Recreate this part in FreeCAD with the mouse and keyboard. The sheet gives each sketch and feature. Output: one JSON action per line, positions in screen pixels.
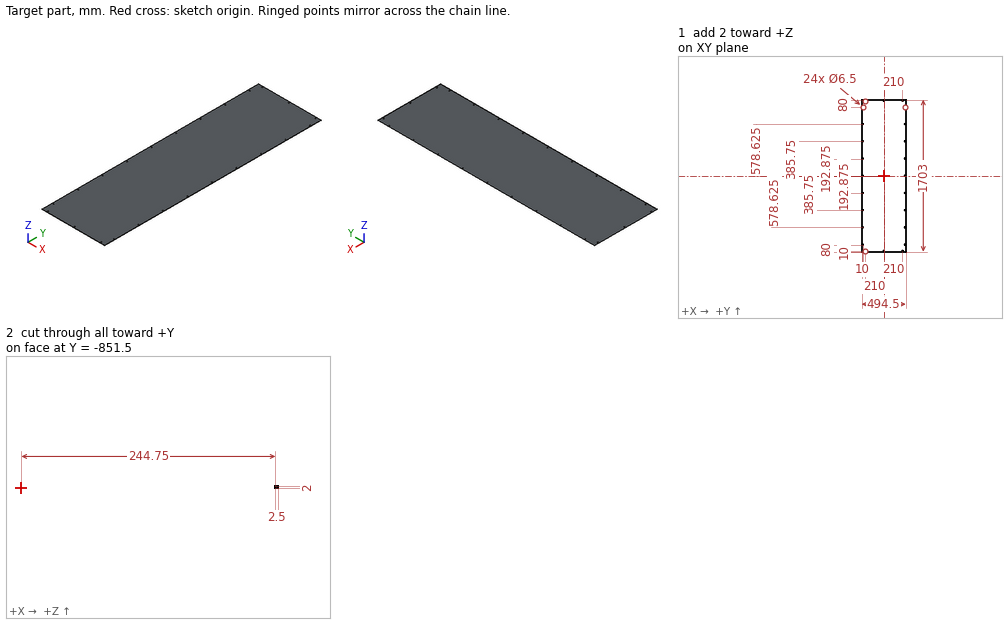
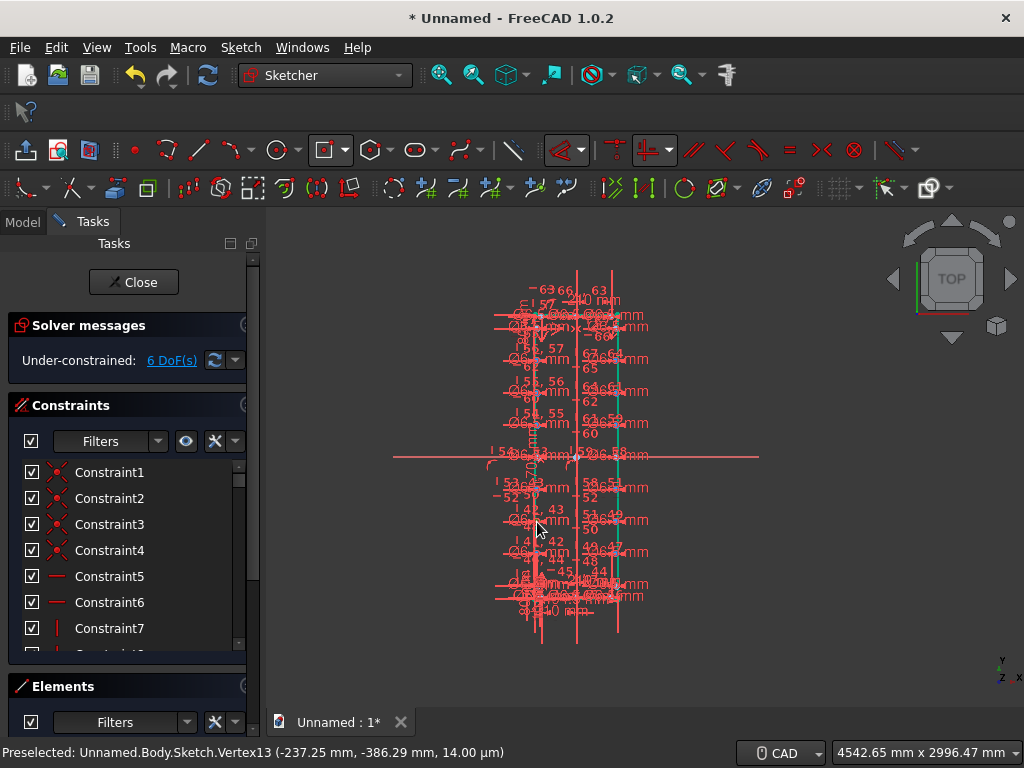
{"action": "left_click", "coordinate": [584, 150]}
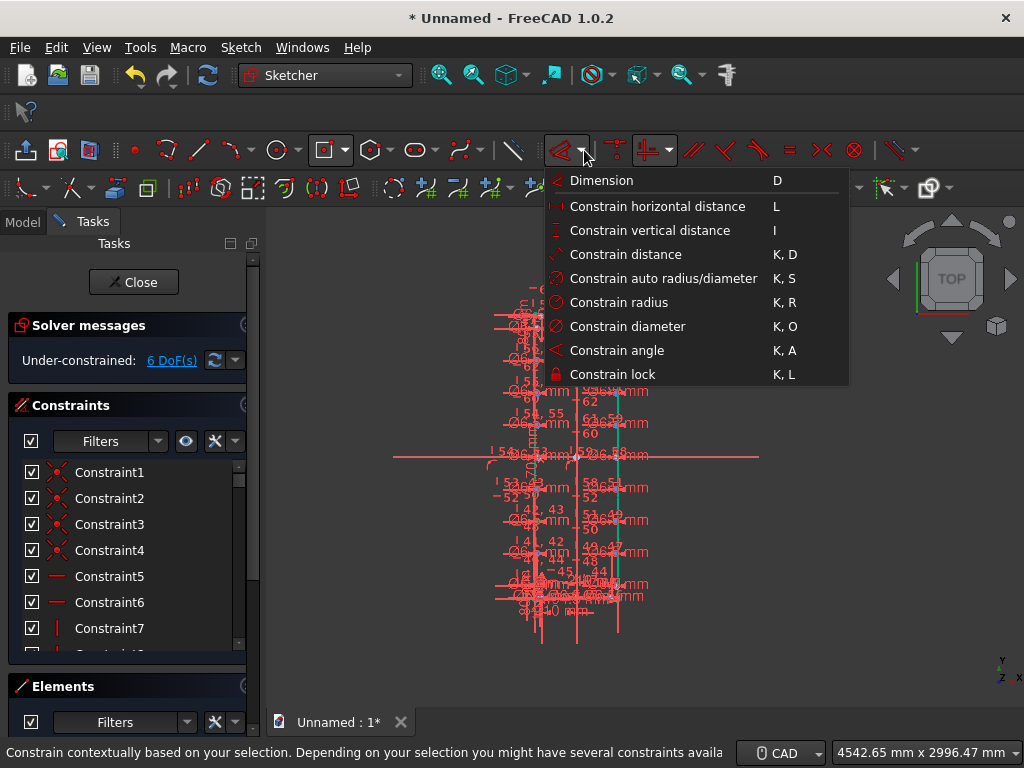
{"action": "left_click", "coordinate": [697, 230]}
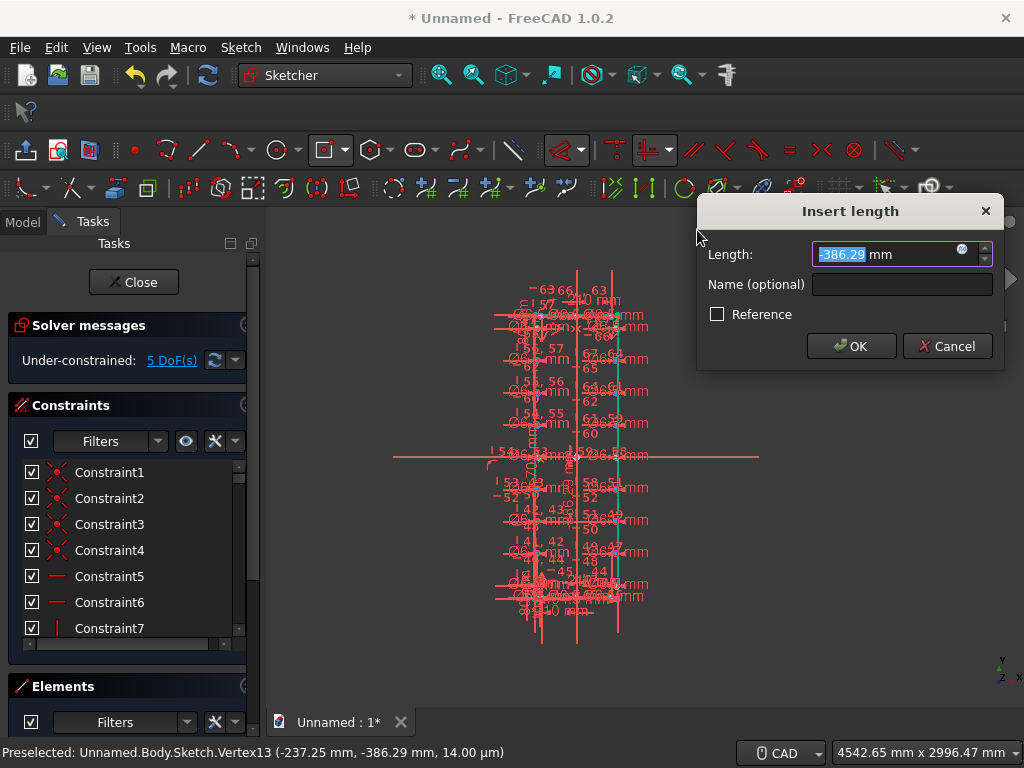
{"action": "type", "text": "-385.75"}
{"action": "key", "text": "Return"}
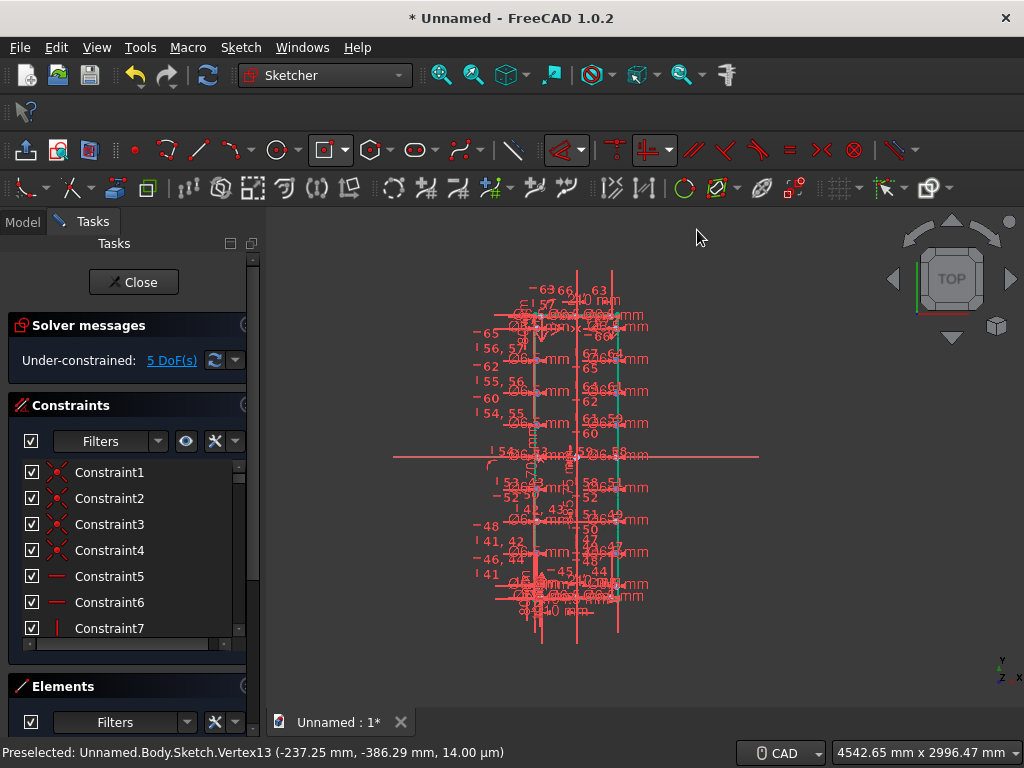
{"action": "left_click", "coordinate": [537, 393]}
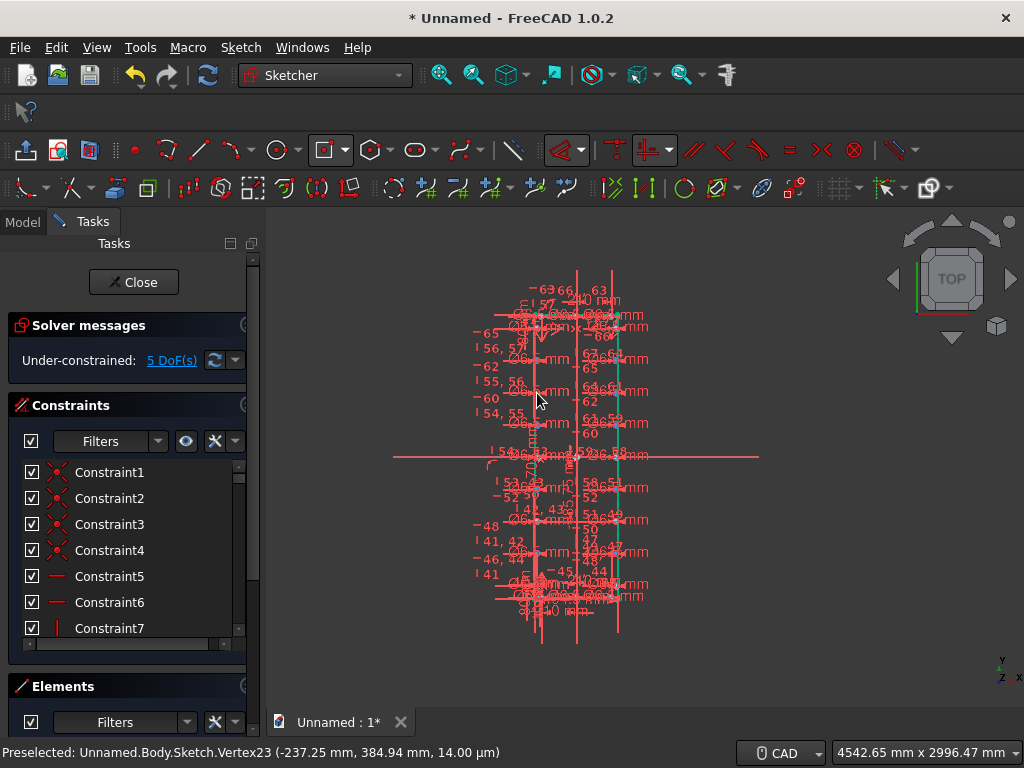
{"action": "key", "text": "i"}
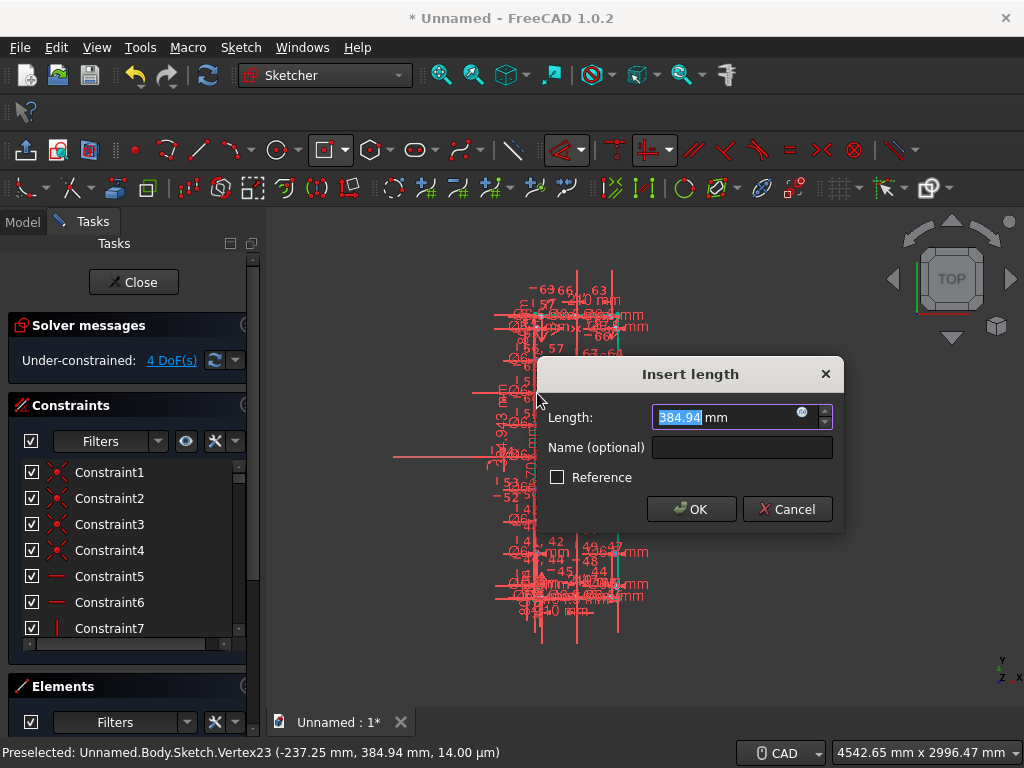
{"action": "type", "text": "385.75"}
{"action": "key", "text": "Return"}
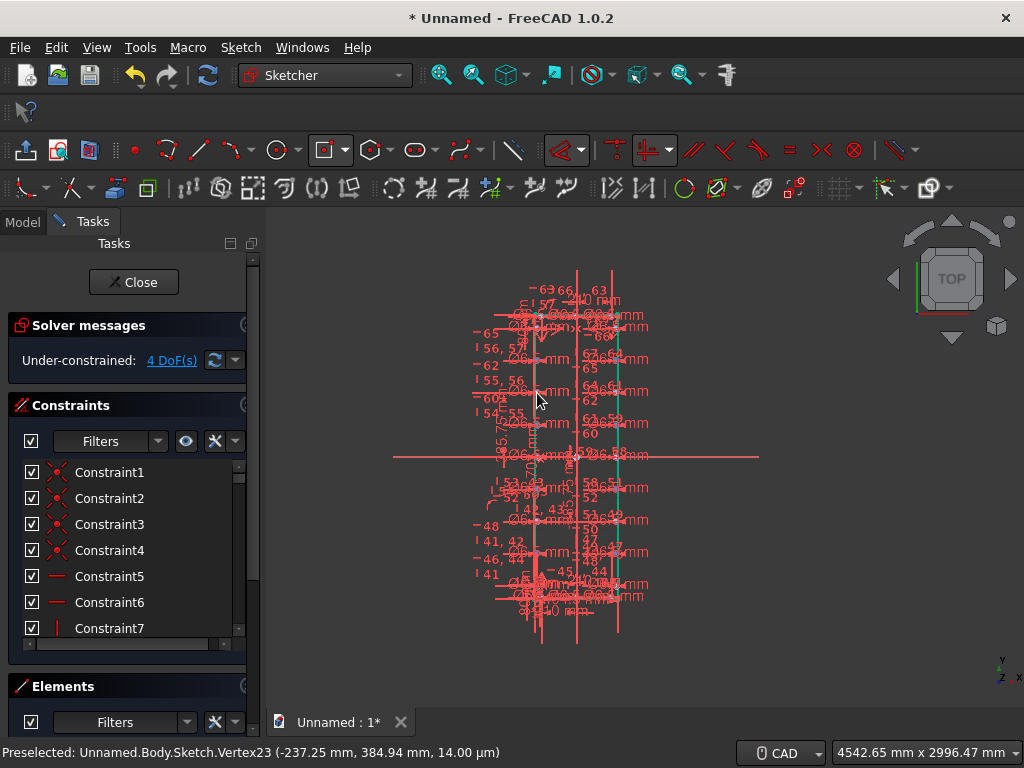
{"action": "left_click", "coordinate": [537, 554]}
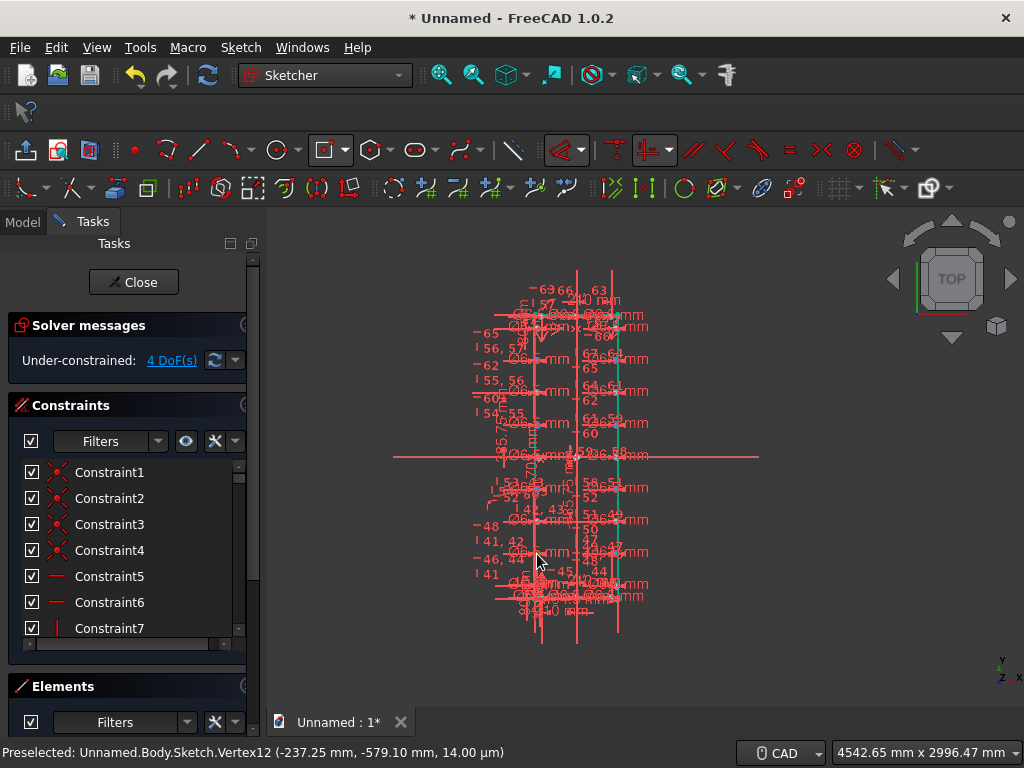
{"action": "key", "text": "i"}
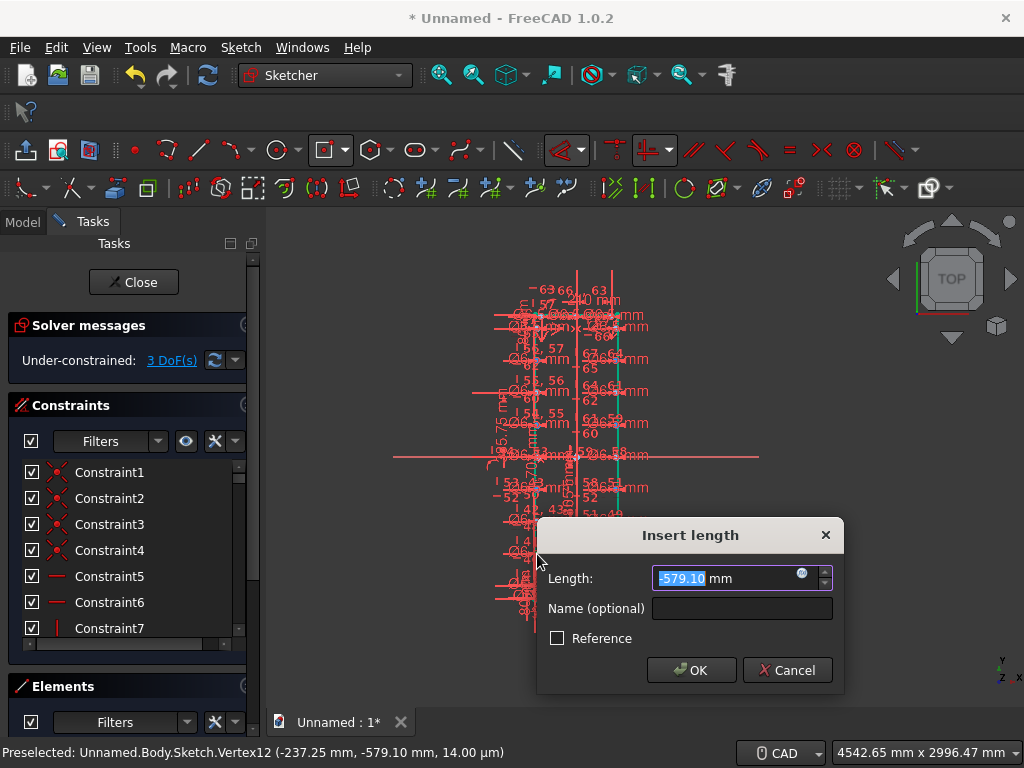
{"action": "type", "text": "-578.625"}
{"action": "key", "text": "Return"}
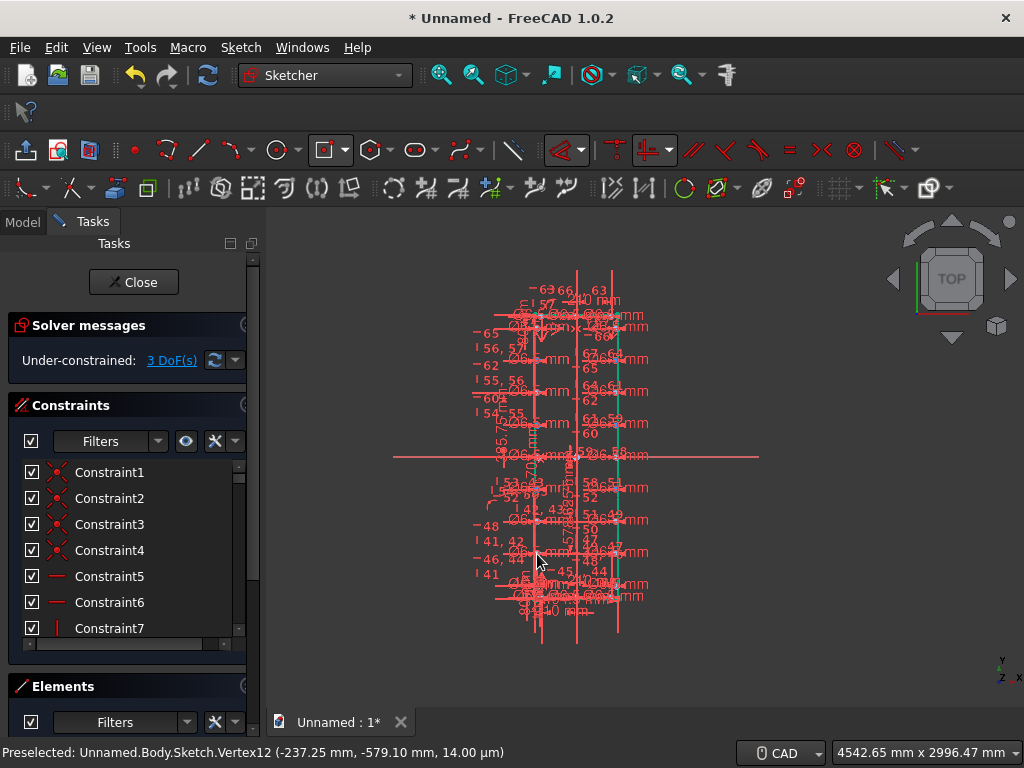
{"action": "scroll", "coordinate": [537, 490], "scroll_direction": "up", "scroll_amount": 2}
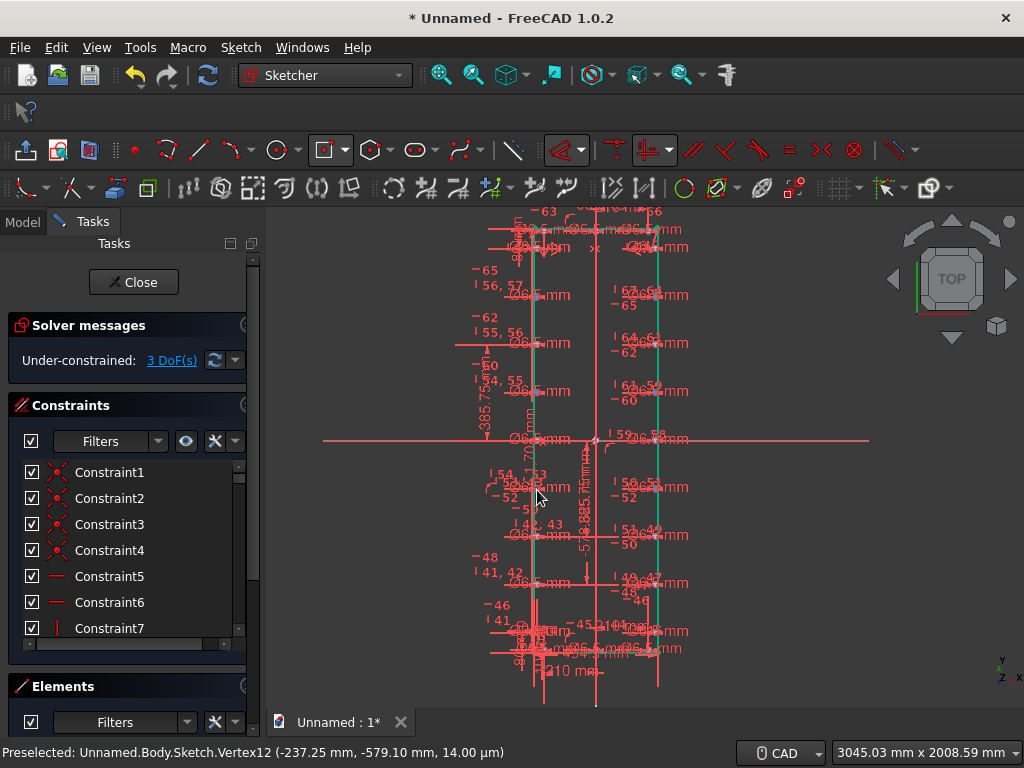
{"action": "left_click", "coordinate": [537, 489]}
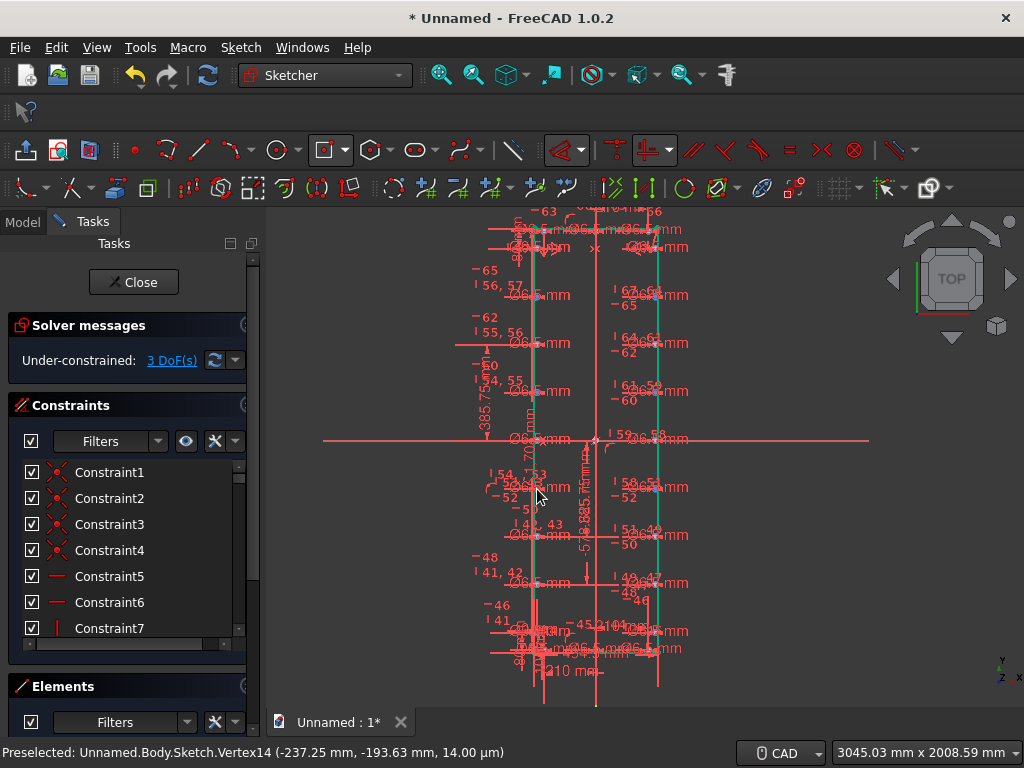
{"action": "left_click", "coordinate": [584, 150]}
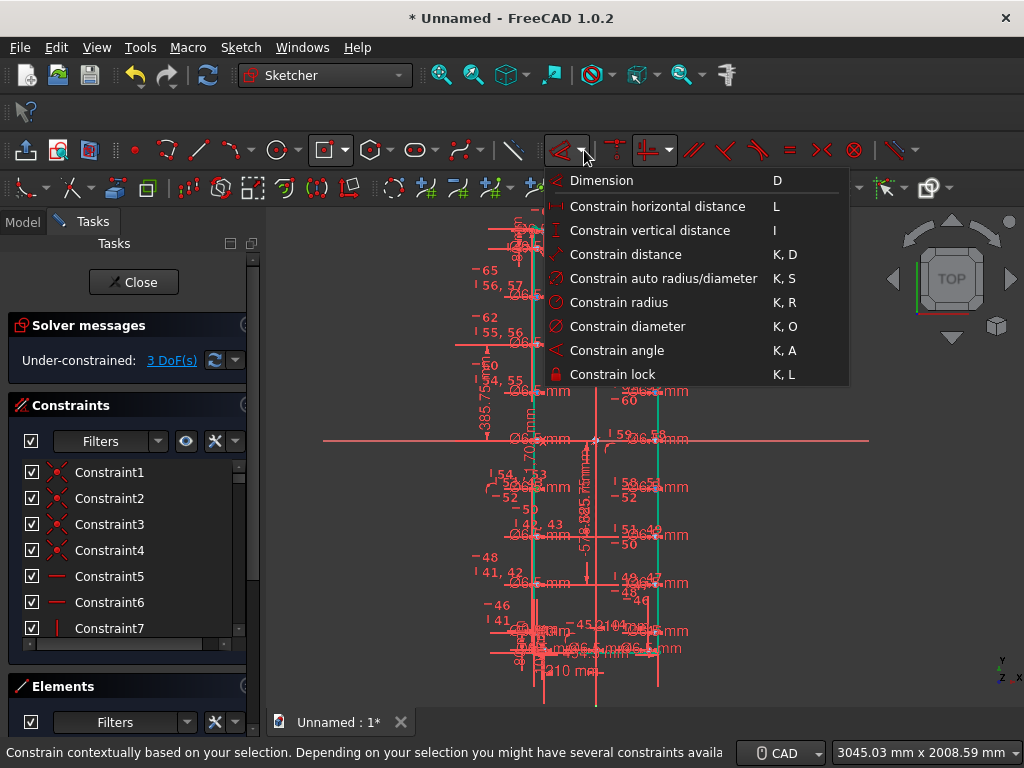
{"action": "left_click", "coordinate": [697, 230]}